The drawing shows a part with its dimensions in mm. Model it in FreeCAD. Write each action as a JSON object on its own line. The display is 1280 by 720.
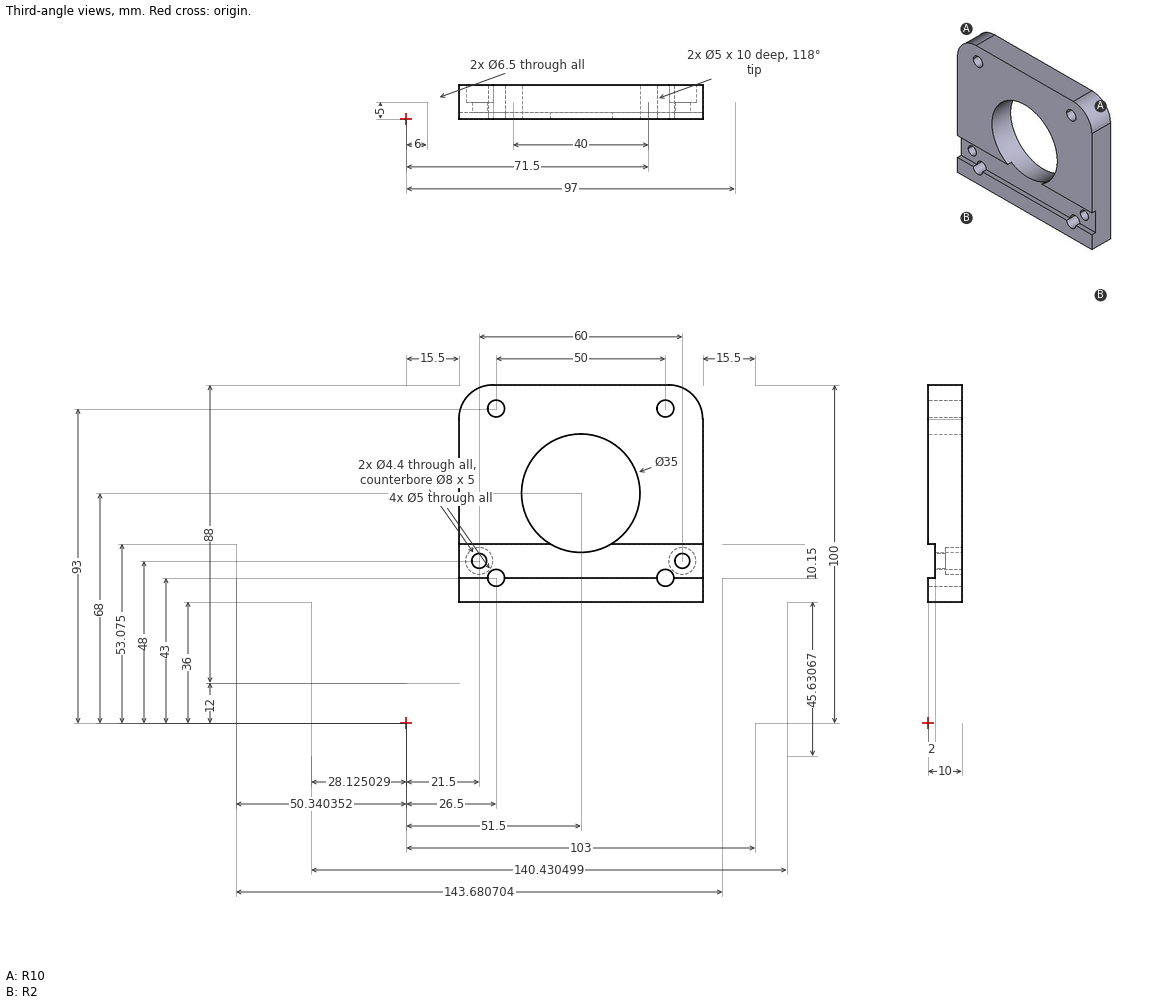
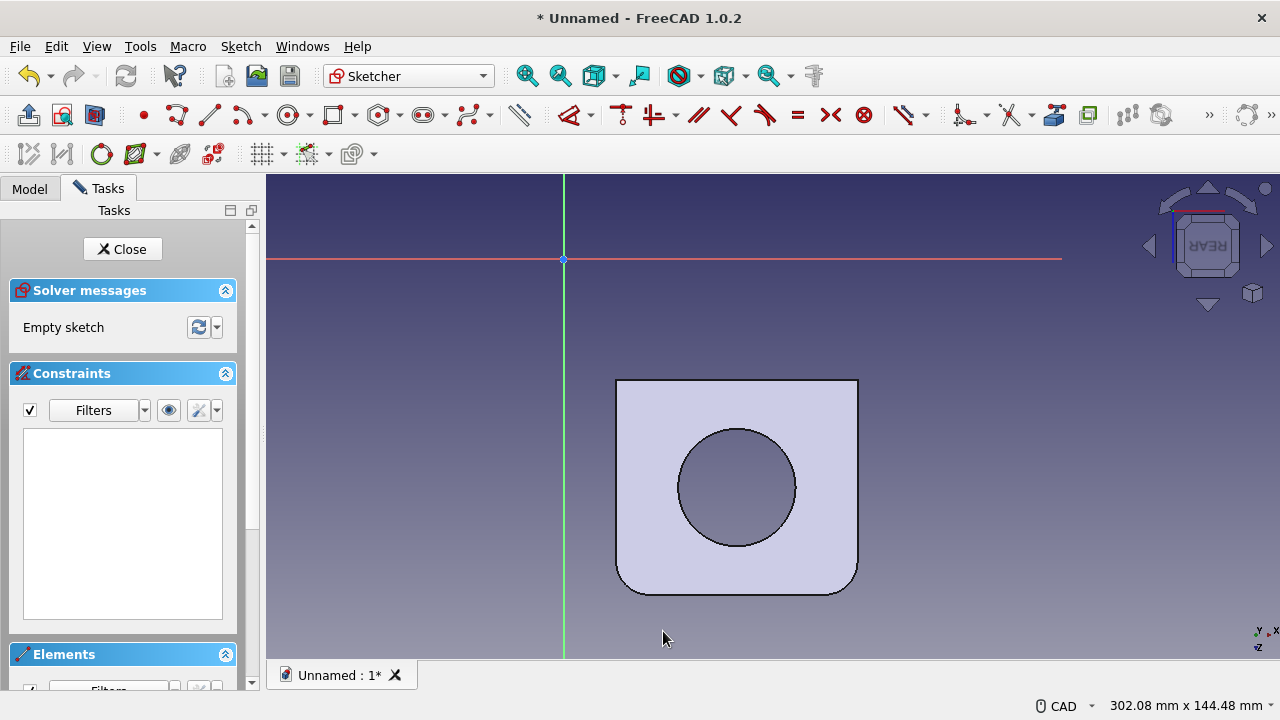
{"action": "scroll", "coordinate": [704, 255], "scroll_direction": "up", "scroll_amount": 3}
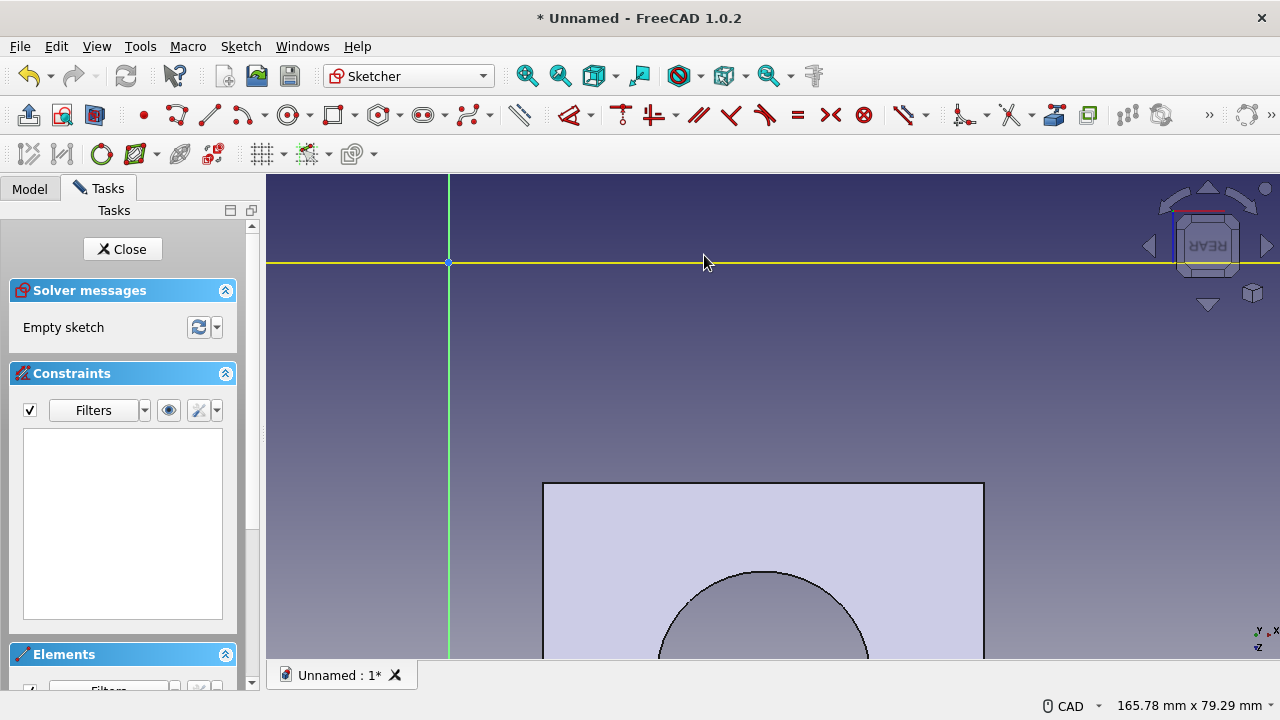
{"action": "key", "text": "g c"}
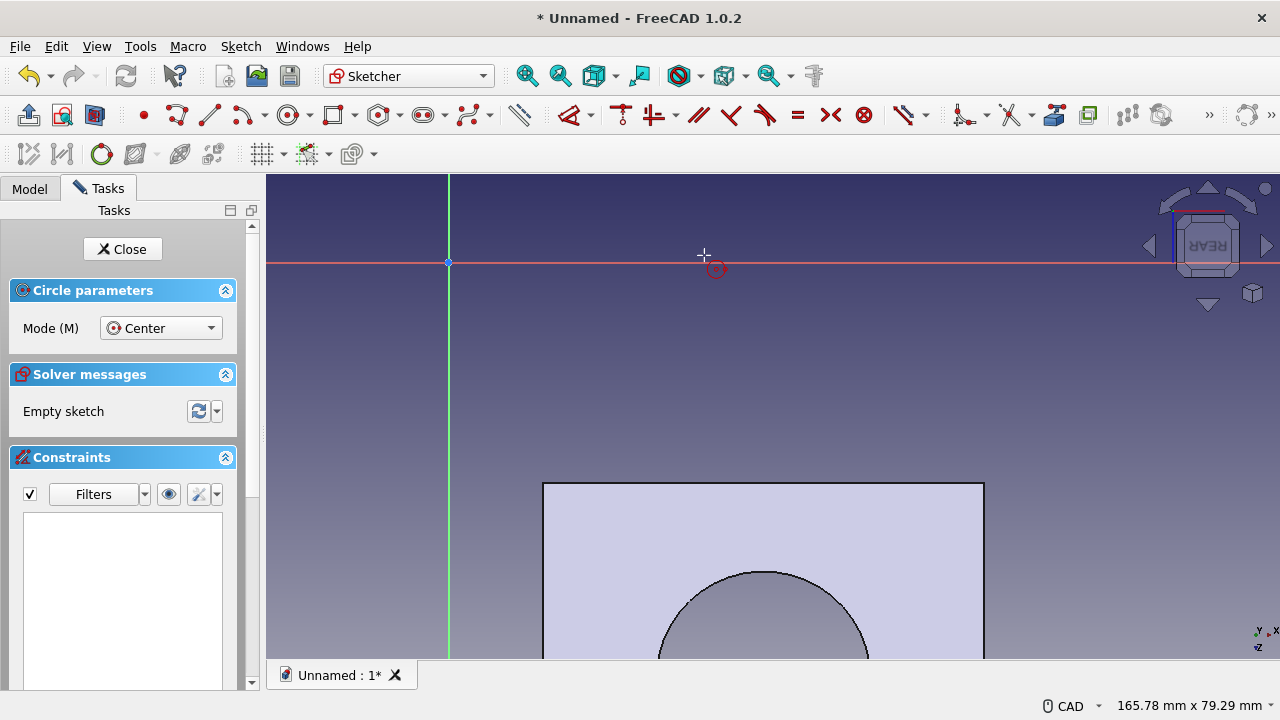
{"action": "scroll", "coordinate": [580, 556], "scroll_direction": "up", "scroll_amount": 3}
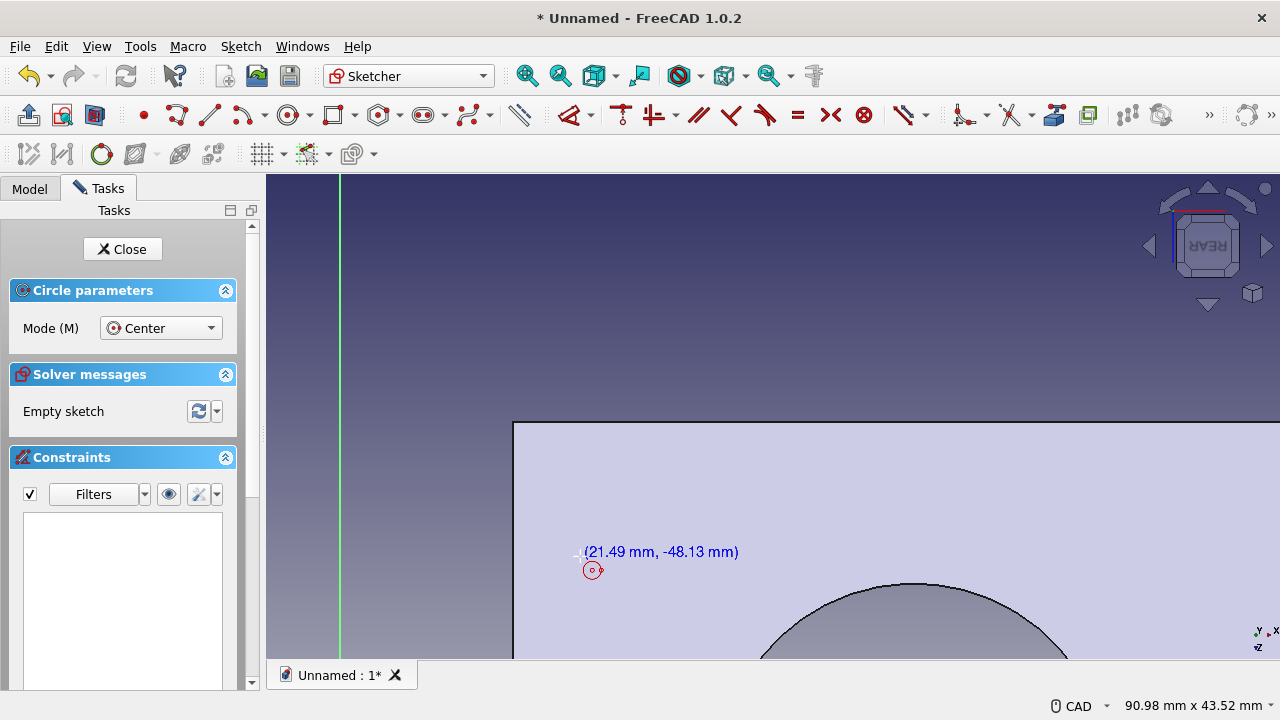
{"action": "left_click", "coordinate": [580, 556]}
{"action": "mouse_move", "coordinate": [597, 538]}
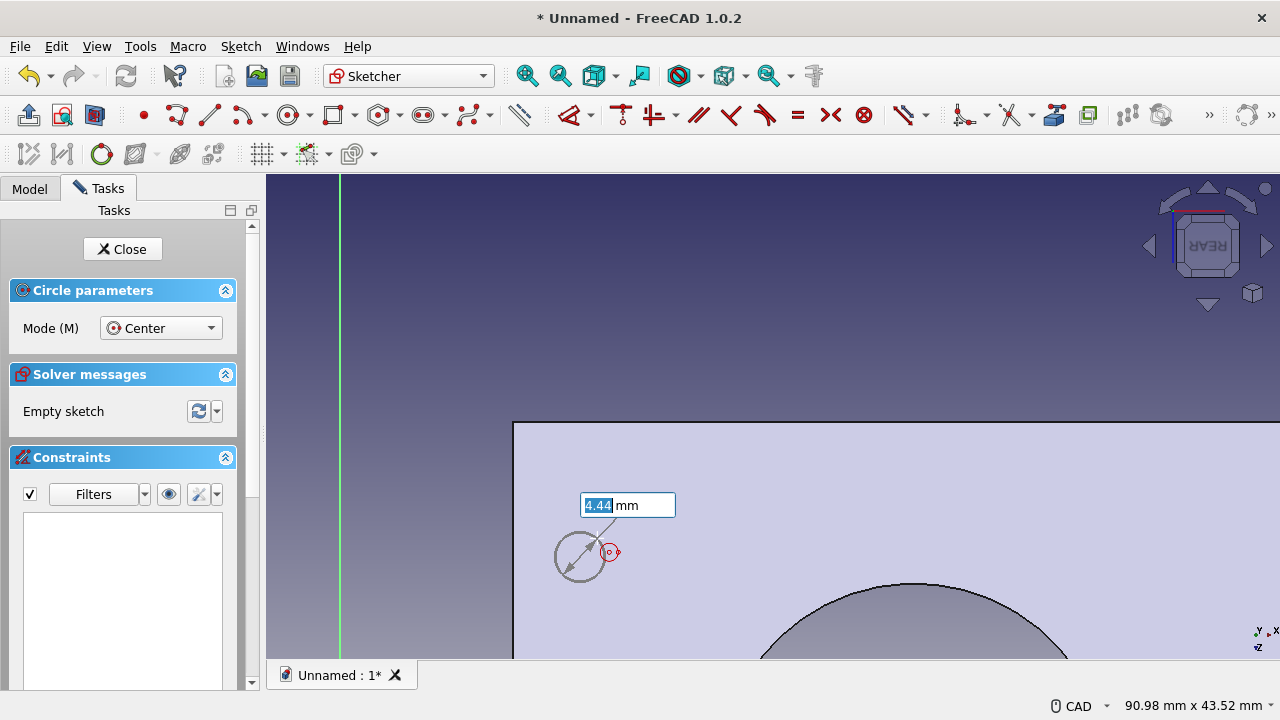
{"action": "type", "text": "4.4"}
{"action": "key", "text": "Return"}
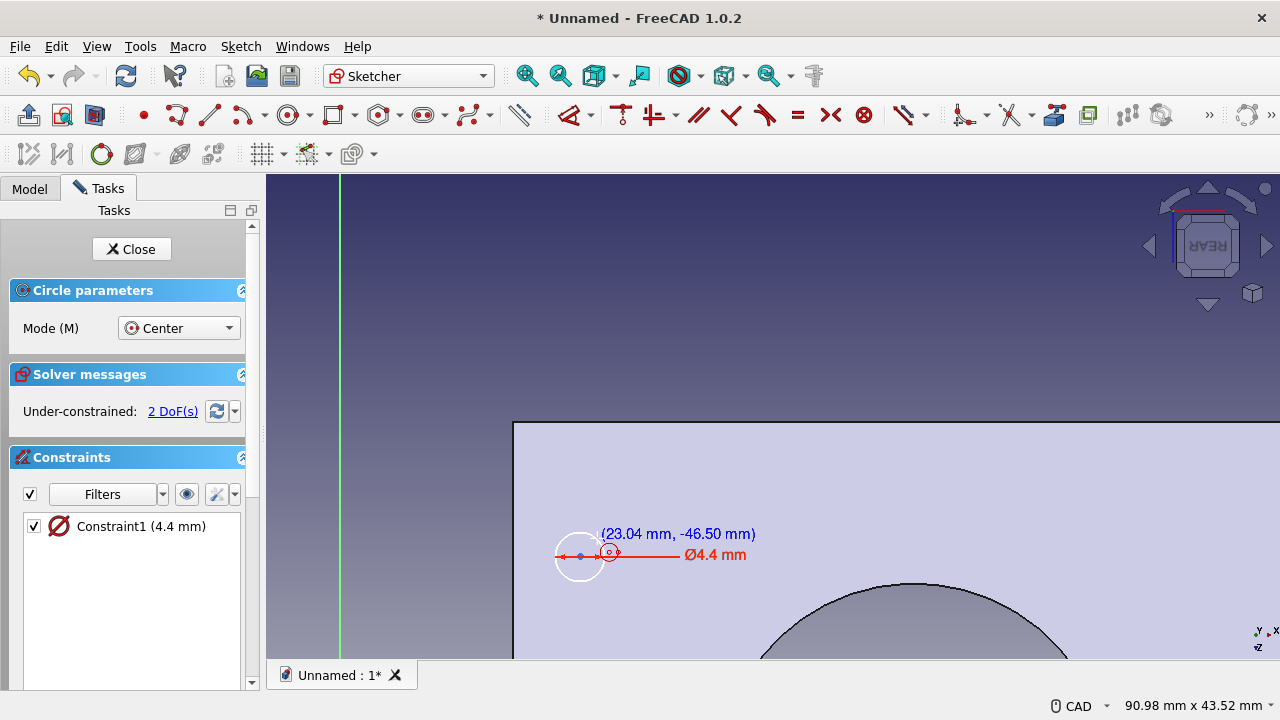
{"action": "scroll", "coordinate": [580, 558], "scroll_direction": "down", "scroll_amount": 3}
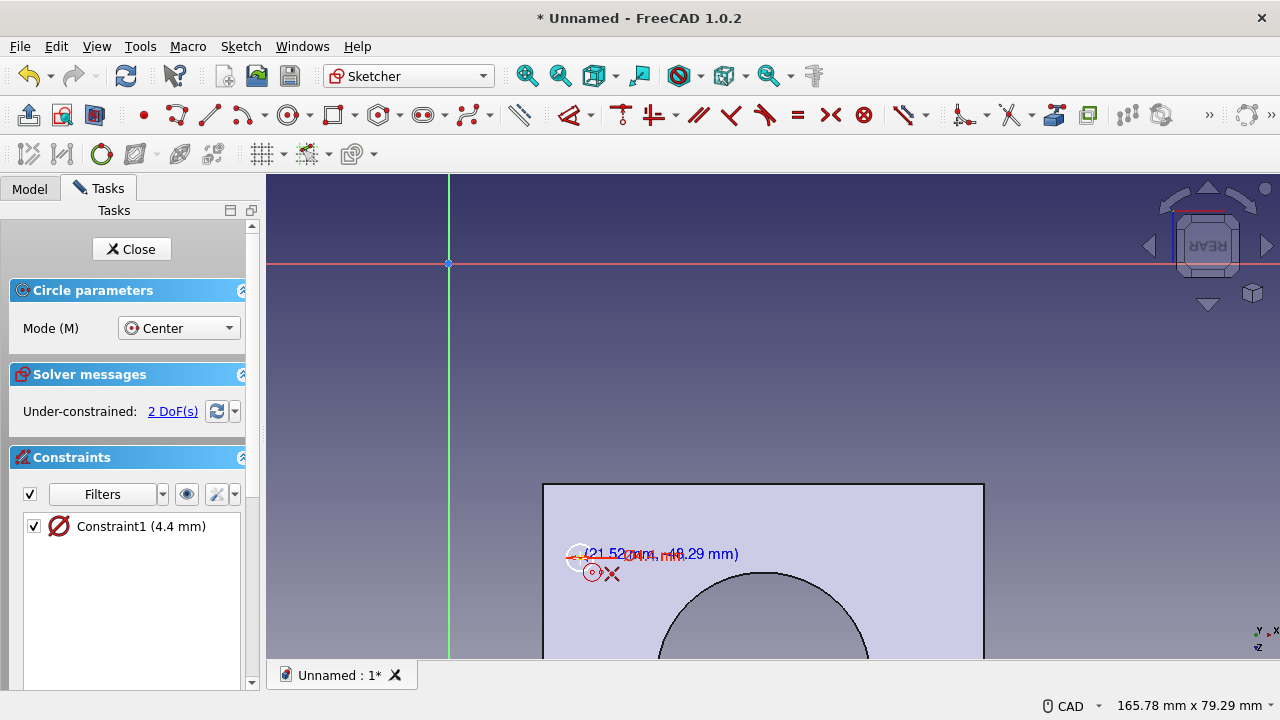
{"action": "scroll", "coordinate": [947, 557], "scroll_direction": "up", "scroll_amount": 3}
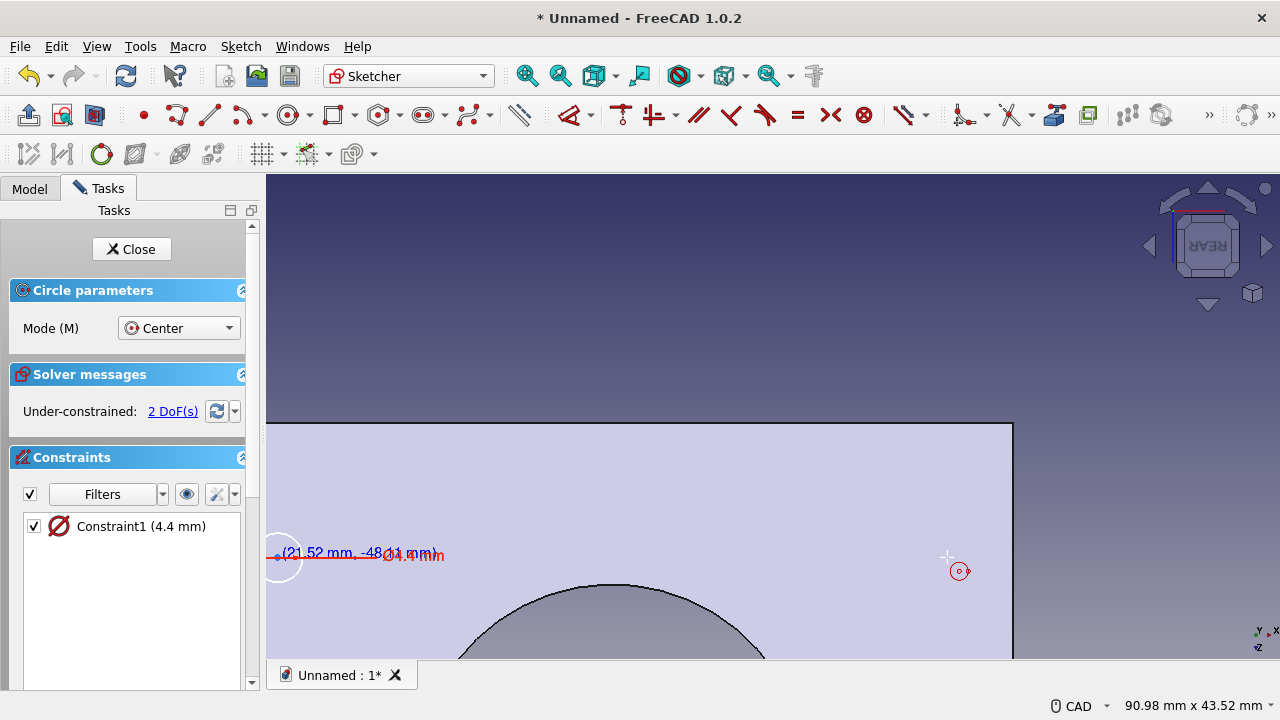
{"action": "left_click", "coordinate": [946, 557]}
{"action": "mouse_move", "coordinate": [964, 539]}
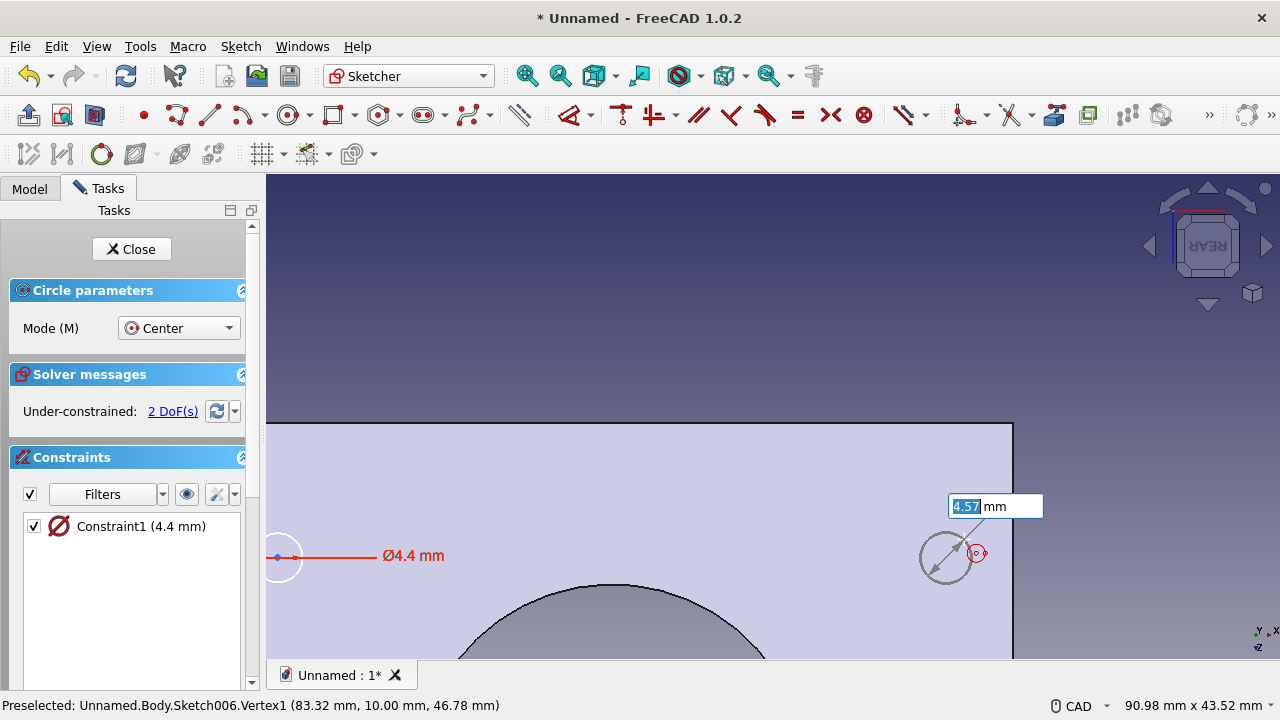
{"action": "type", "text": "4.4"}
{"action": "key", "text": "Return"}
{"action": "key", "text": "Escape"}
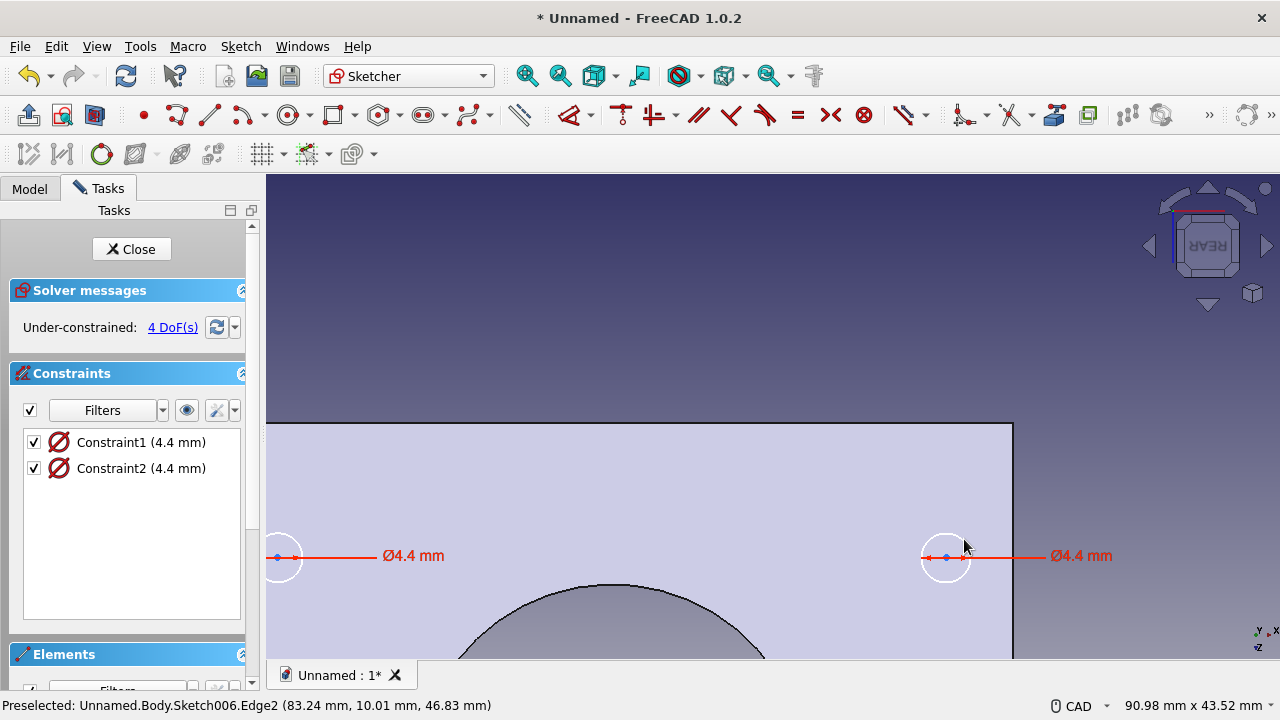
{"action": "left_click", "coordinate": [568, 116]}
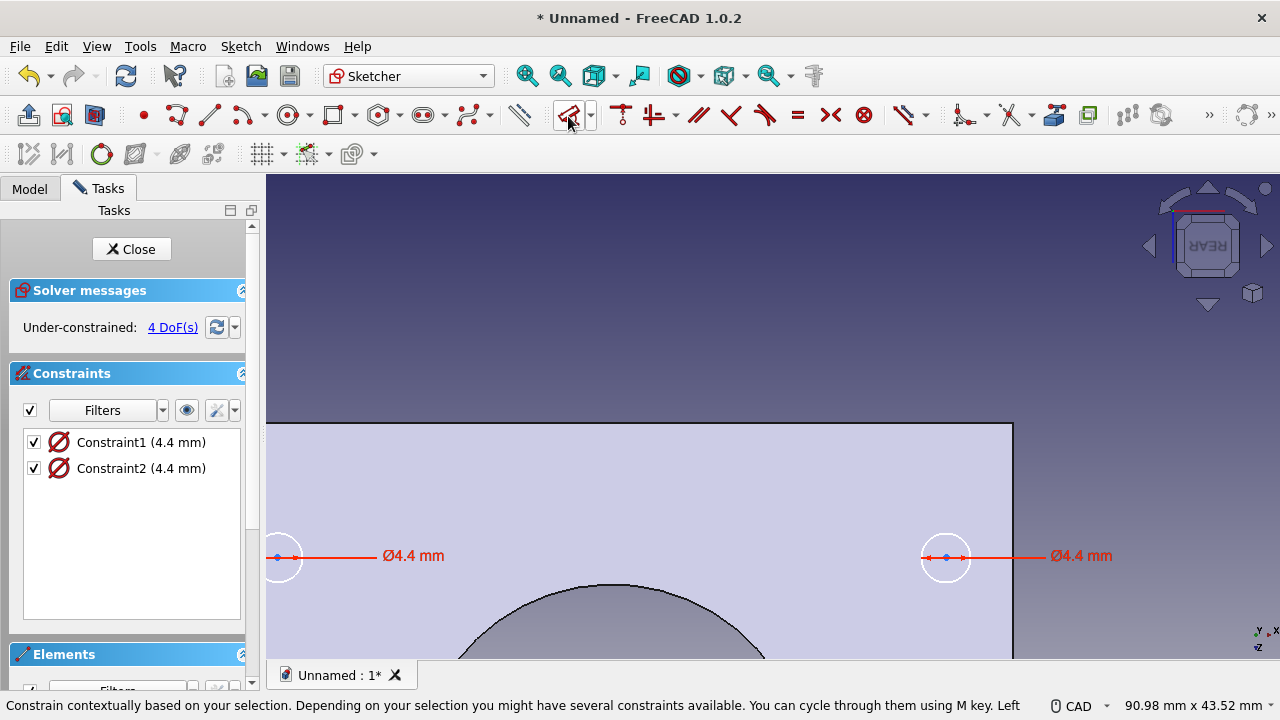
{"action": "scroll", "coordinate": [948, 557], "scroll_direction": "down", "scroll_amount": 3}